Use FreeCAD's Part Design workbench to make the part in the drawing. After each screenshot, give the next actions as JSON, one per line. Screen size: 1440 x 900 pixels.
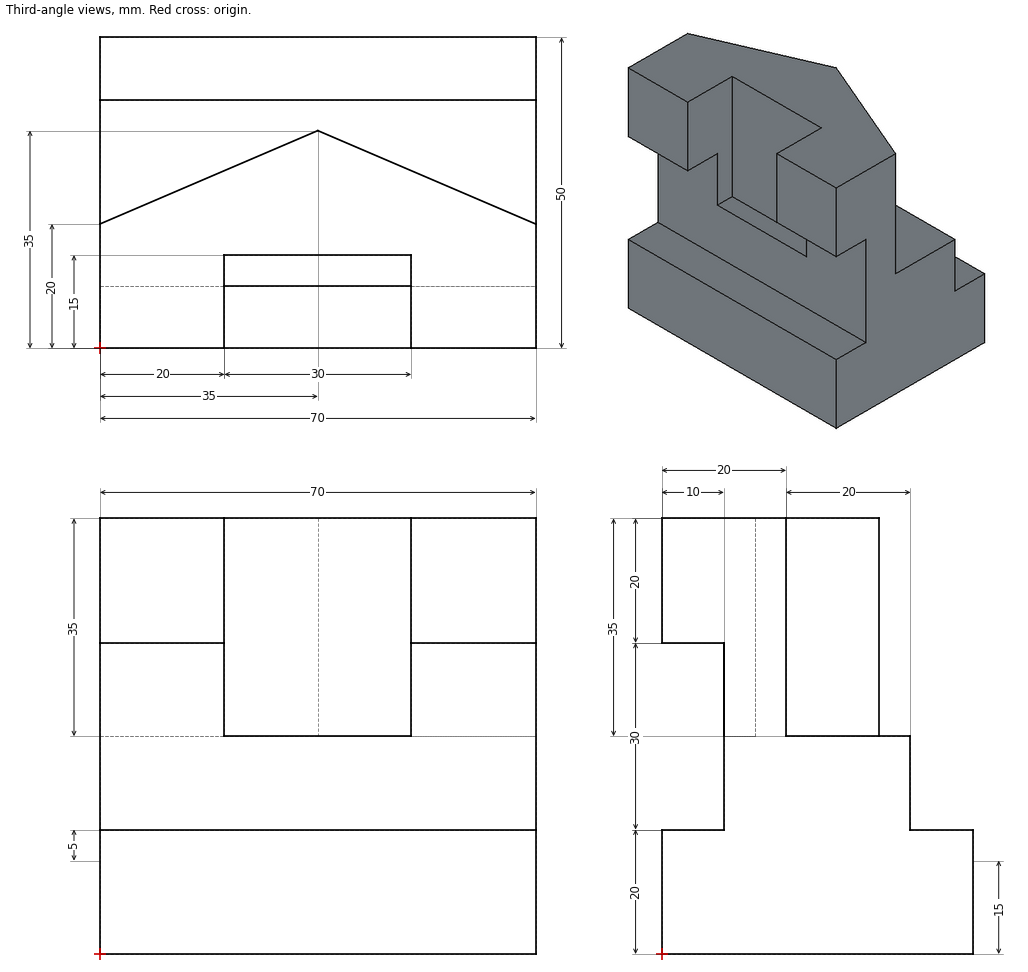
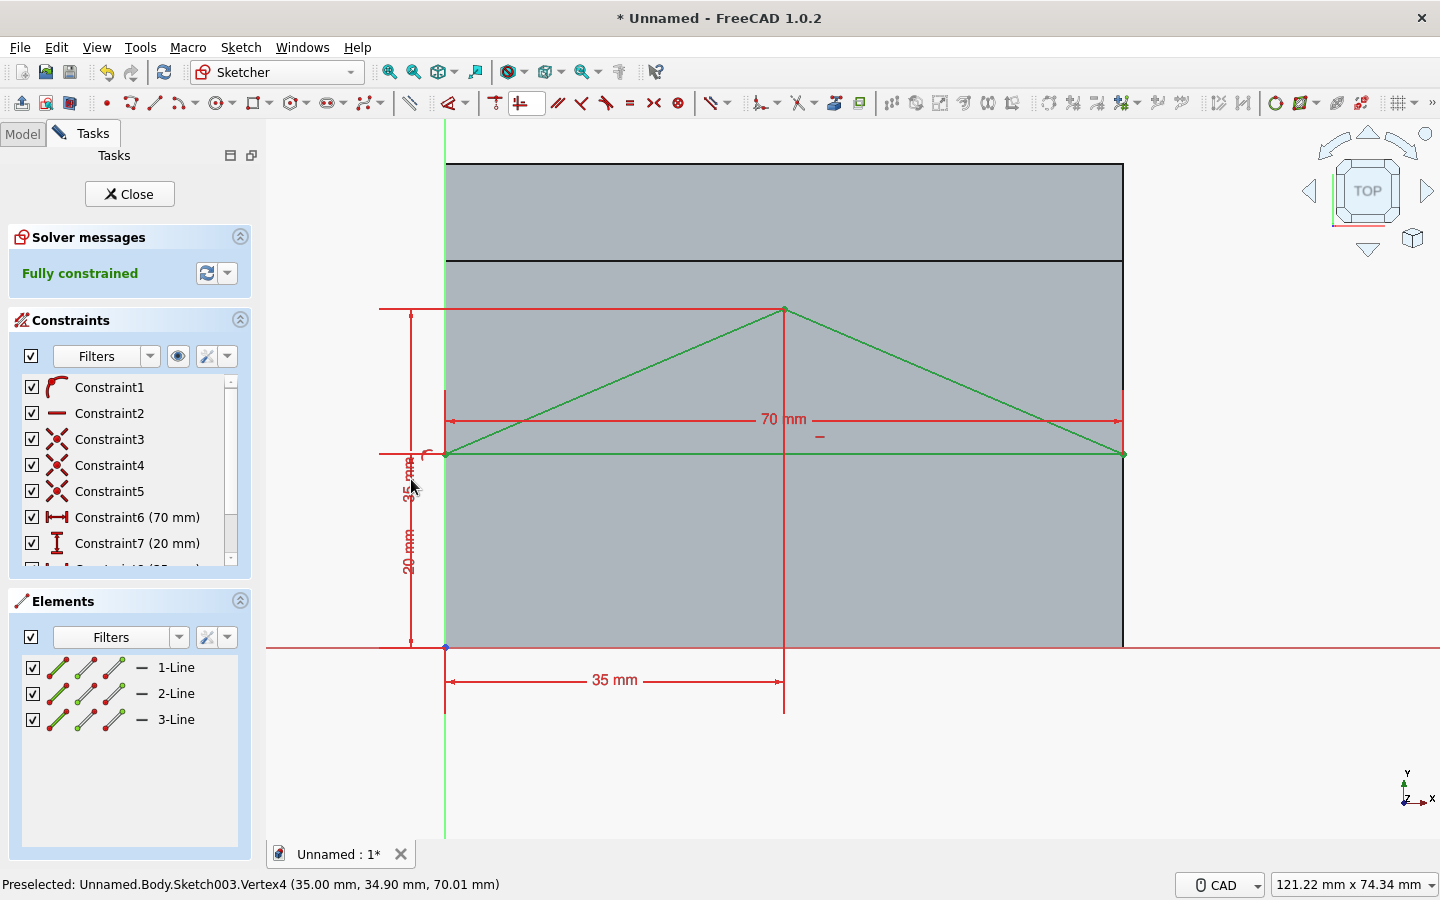
{"action": "left_click", "coordinate": [130, 194]}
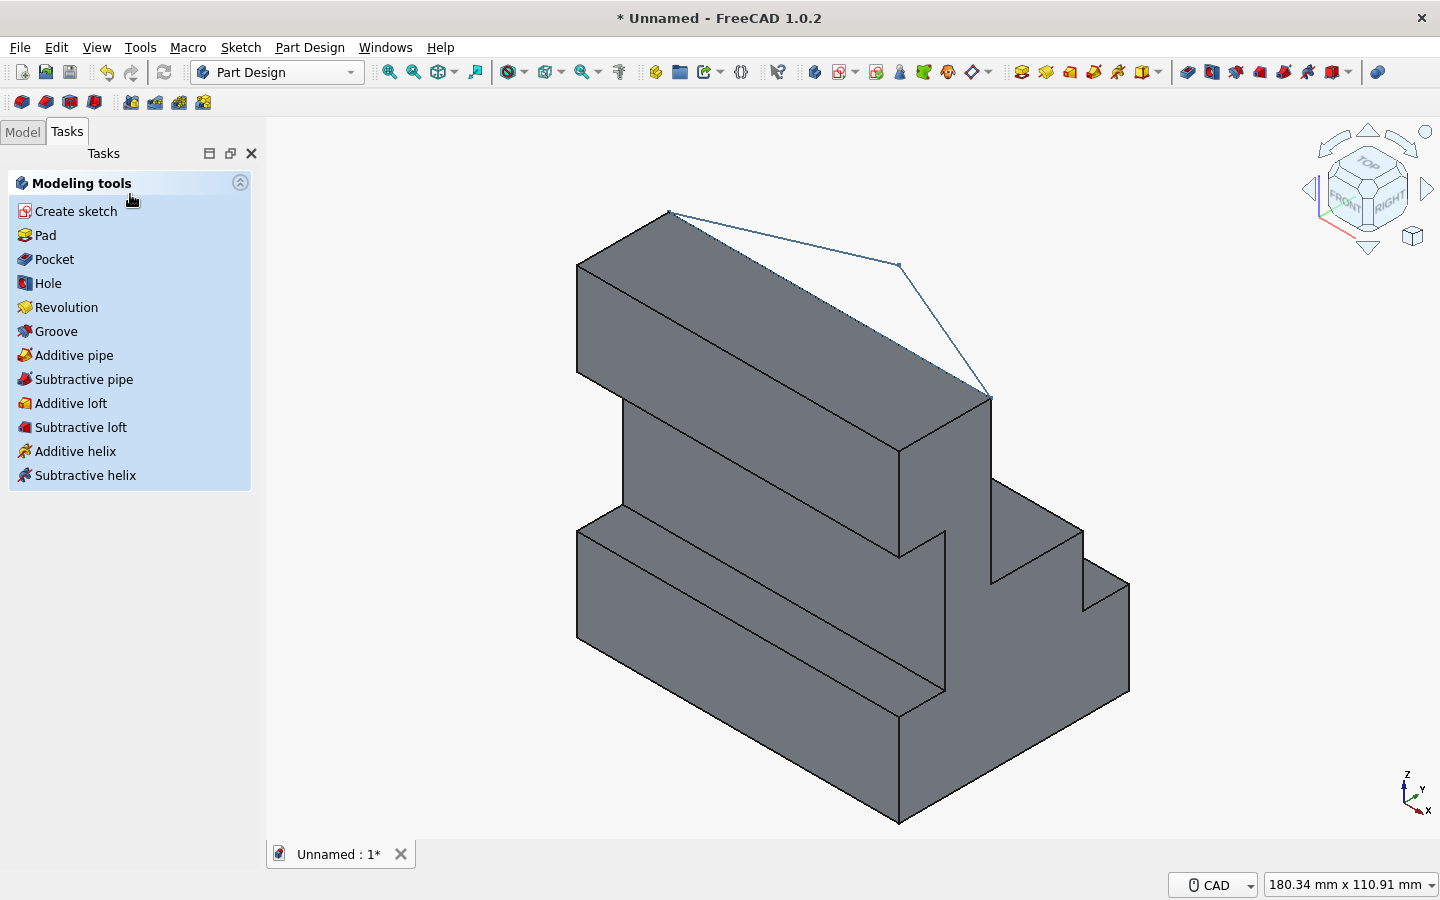
{"action": "left_click", "coordinate": [1022, 72]}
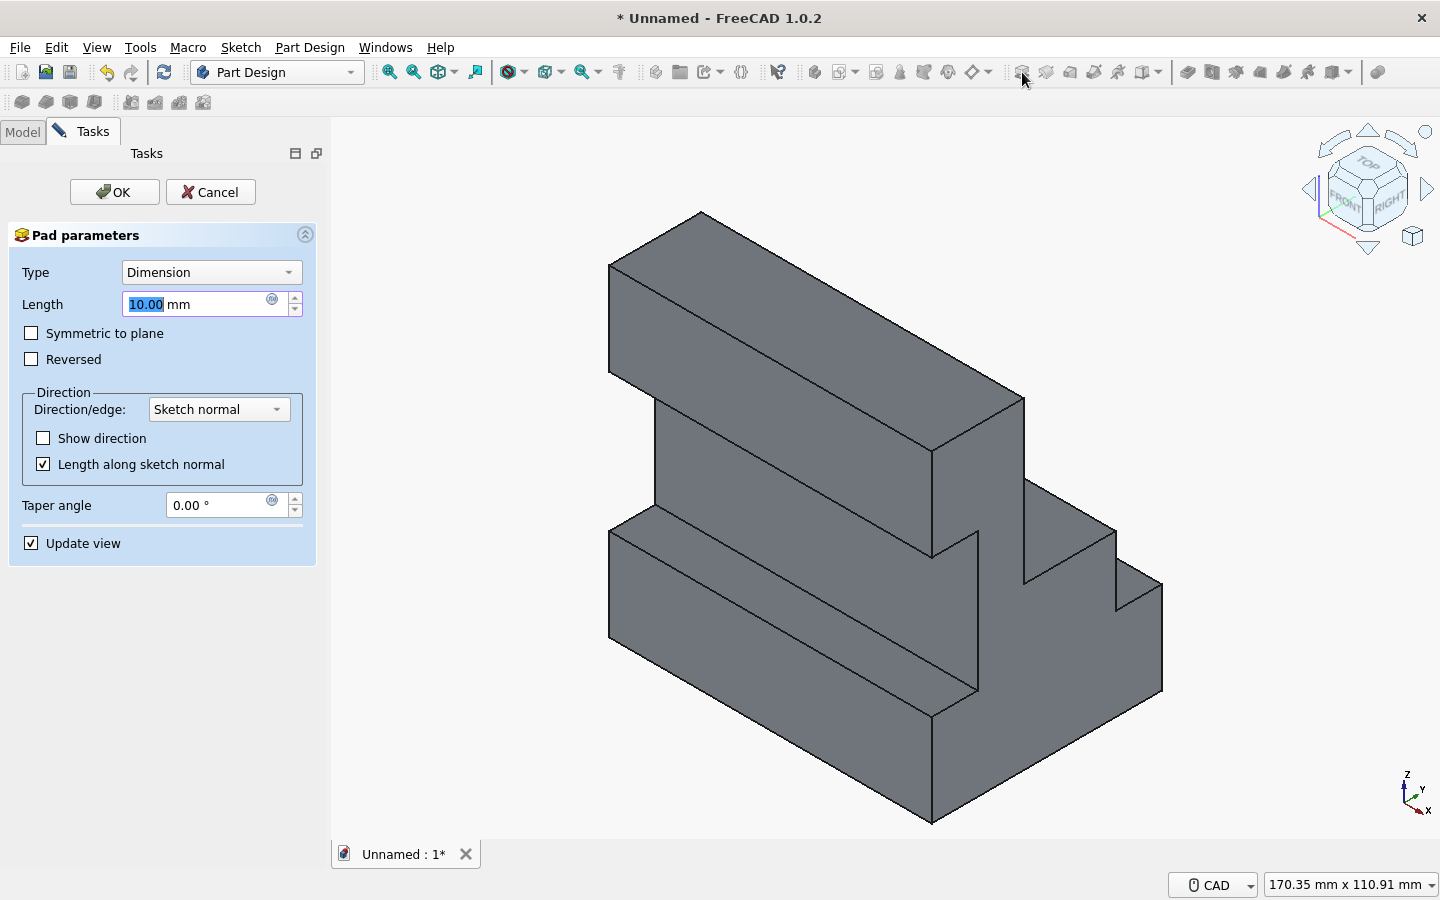
{"action": "type", "text": "35"}
{"action": "key", "text": "Tab"}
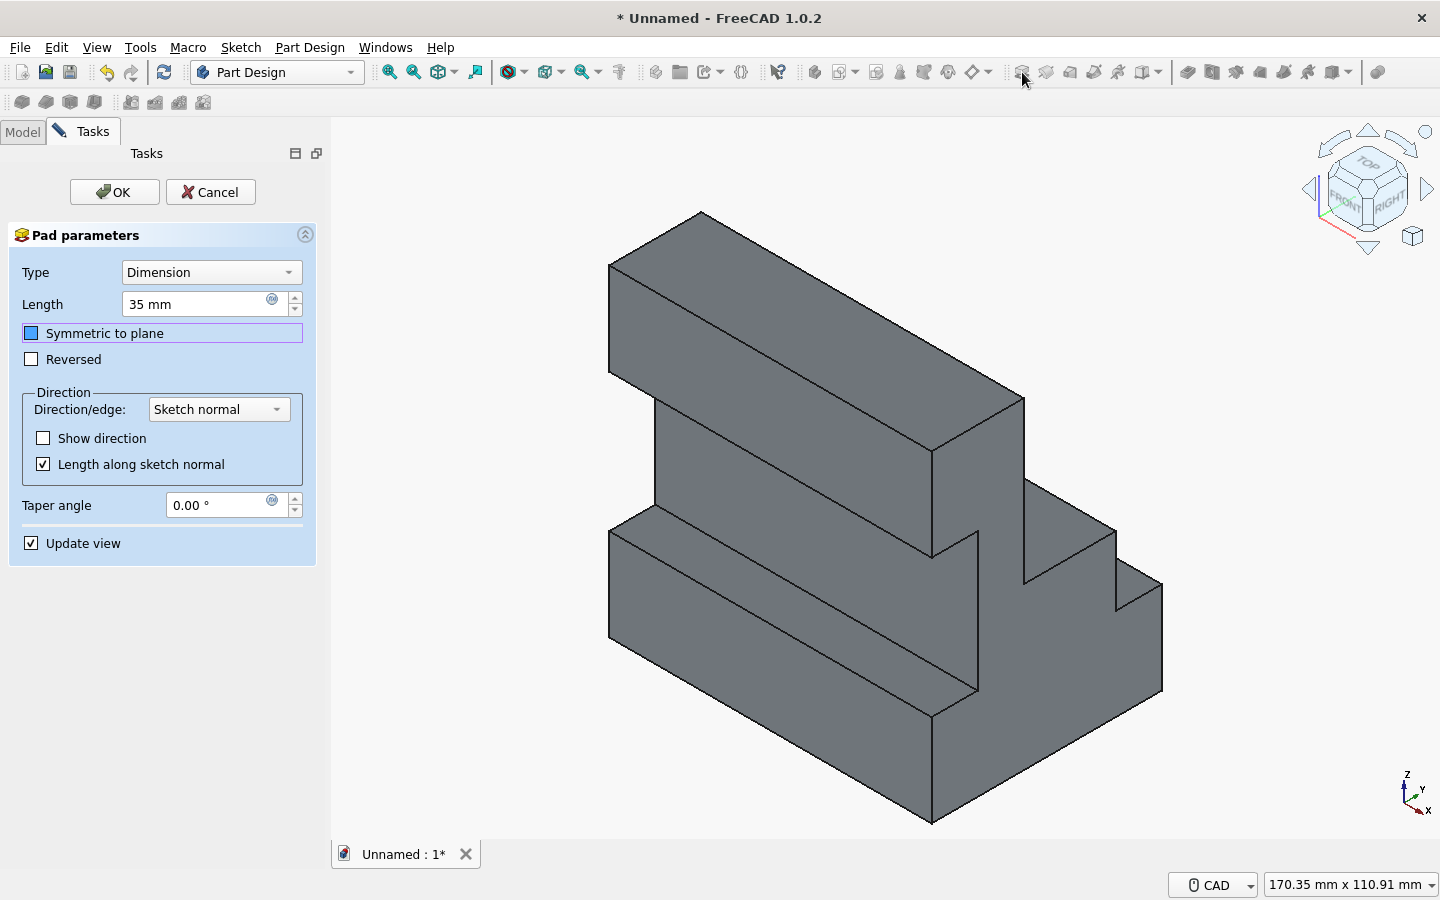
{"action": "left_click", "coordinate": [30, 359]}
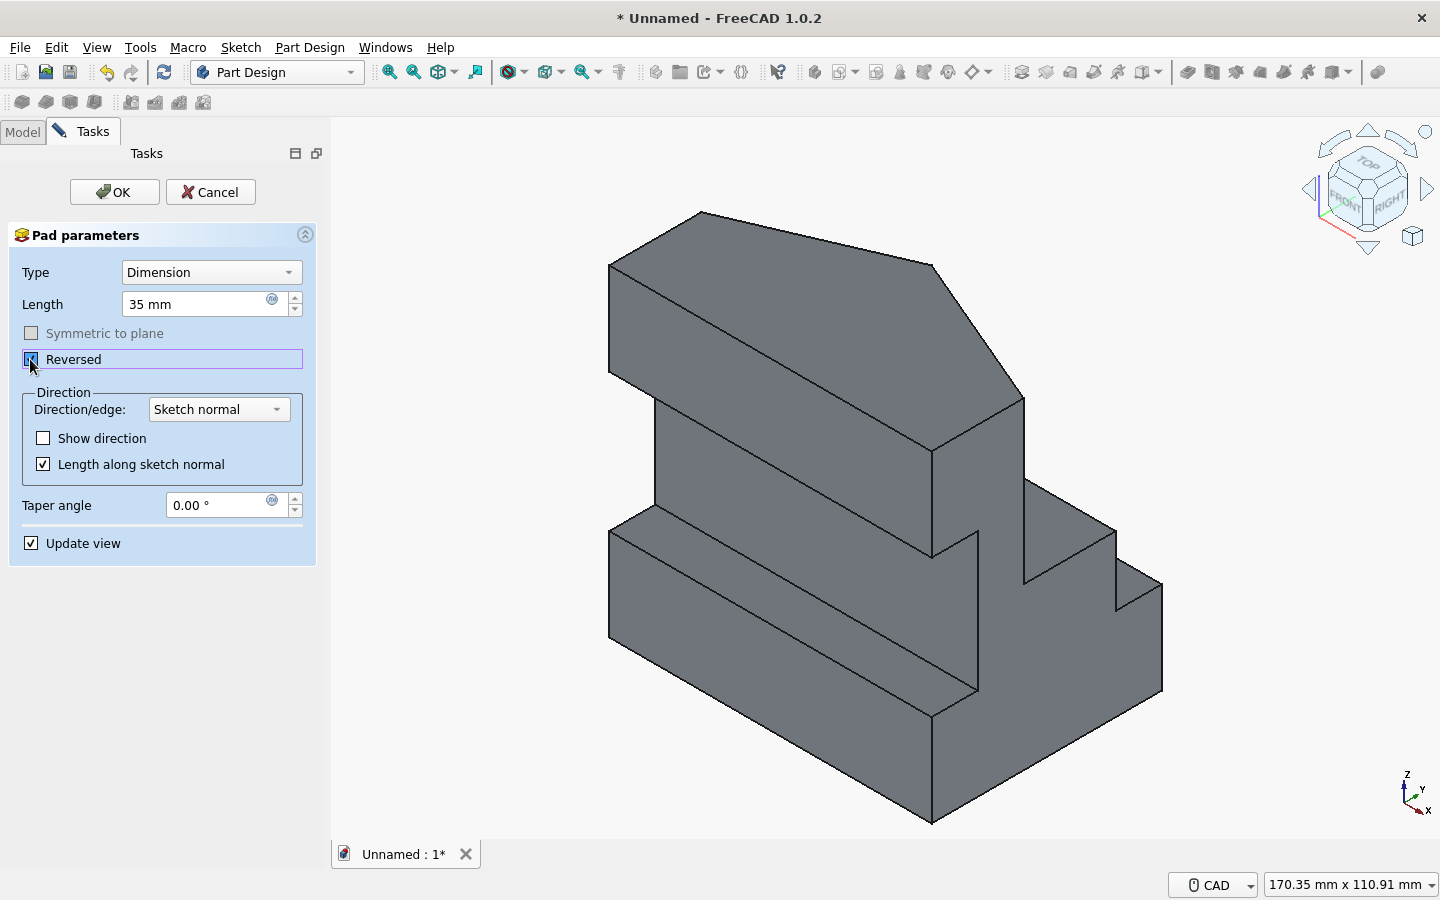
{"action": "left_click", "coordinate": [115, 192]}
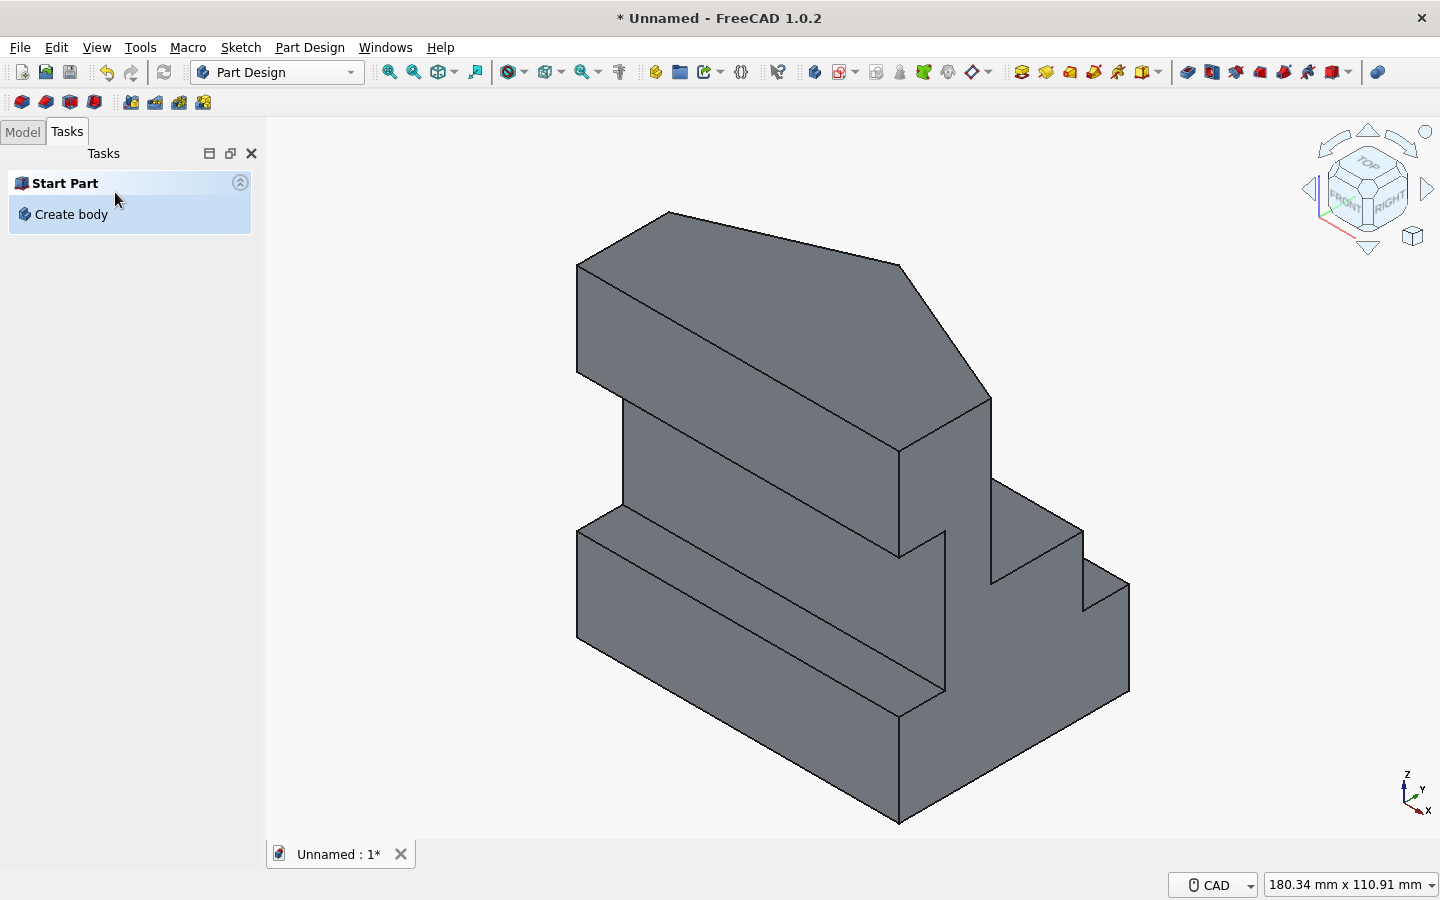
{"action": "left_click", "coordinate": [818, 311]}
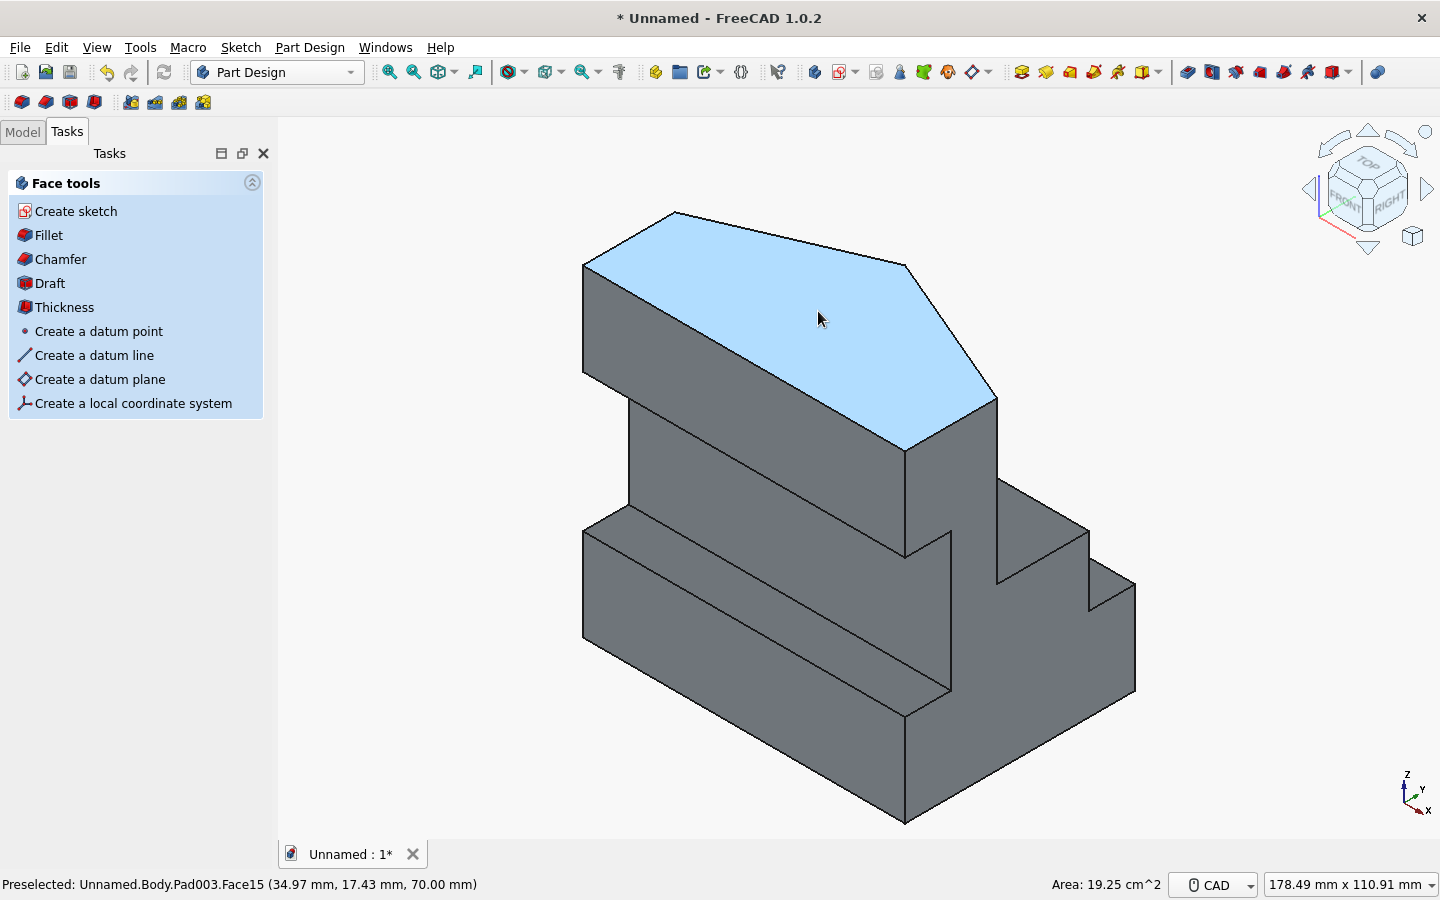
{"action": "left_click", "coordinate": [840, 72]}